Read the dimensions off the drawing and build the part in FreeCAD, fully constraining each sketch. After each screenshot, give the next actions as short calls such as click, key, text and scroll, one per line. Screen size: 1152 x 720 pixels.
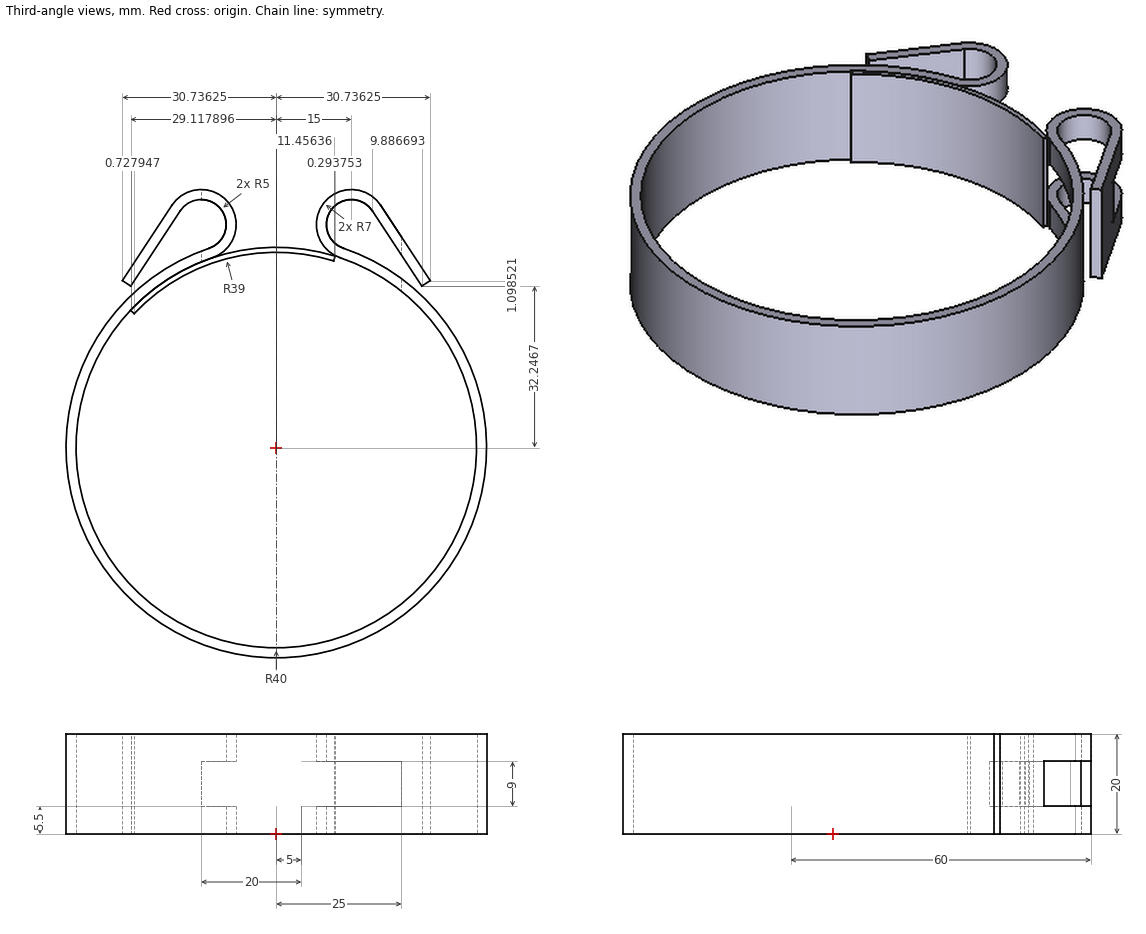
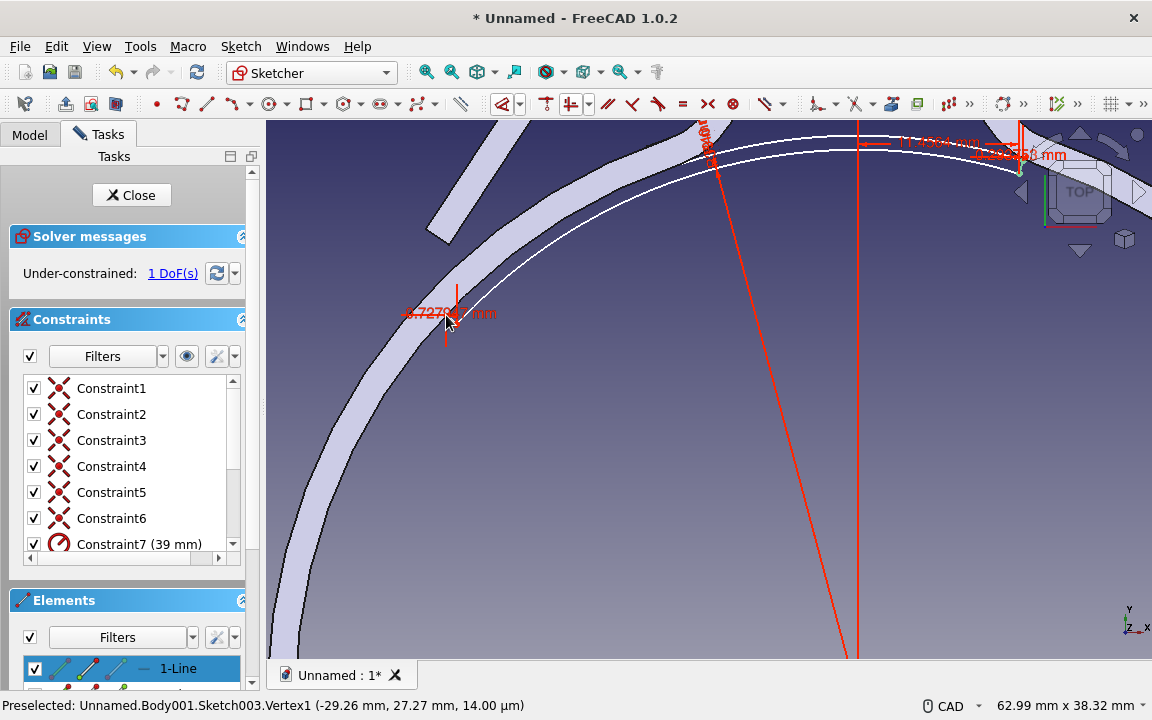
key(l)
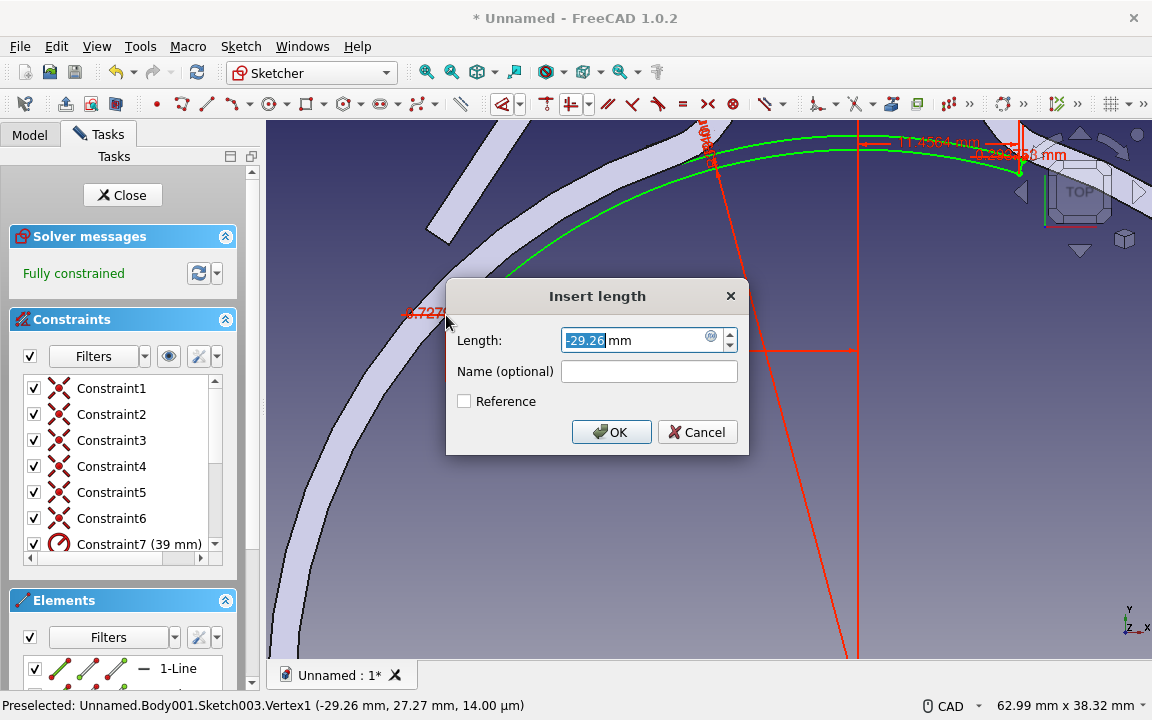
text(-29.117896)
key(Return)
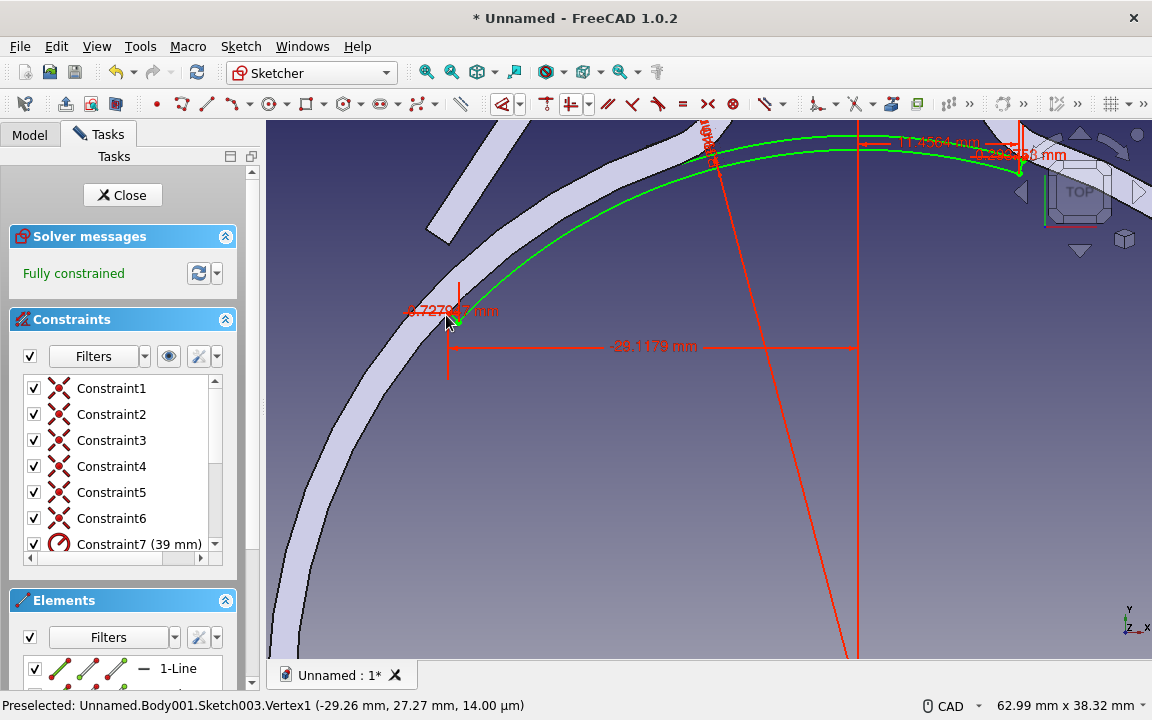
click(123, 195)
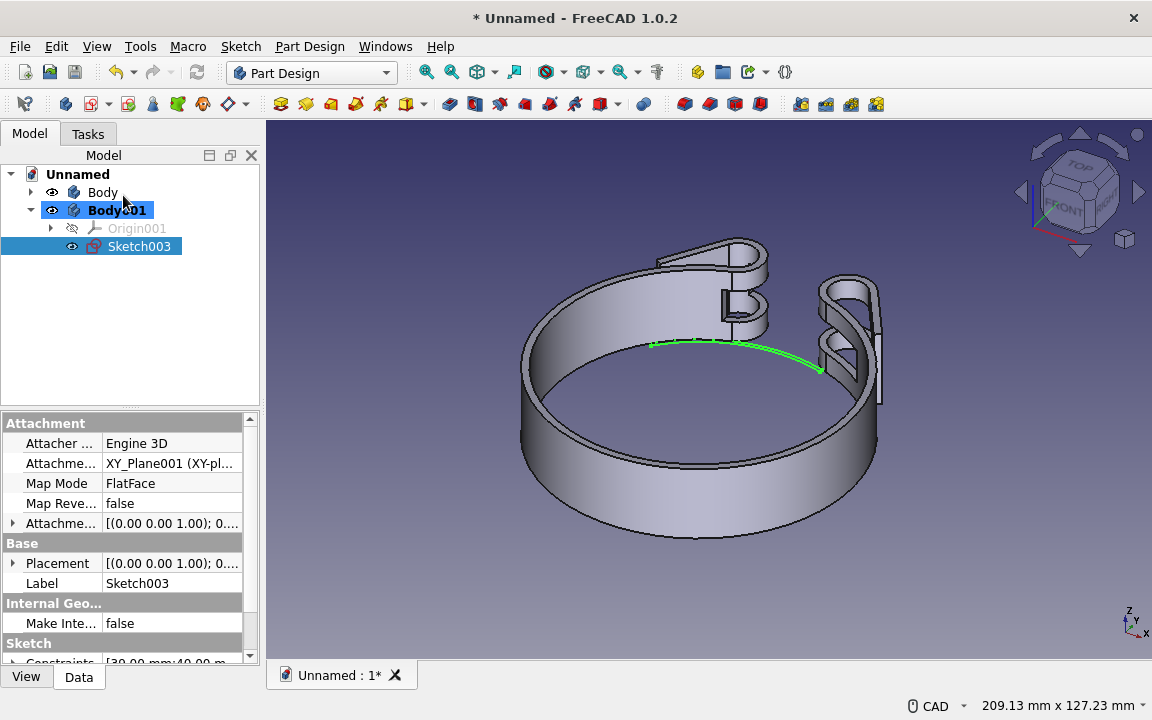
click(281, 104)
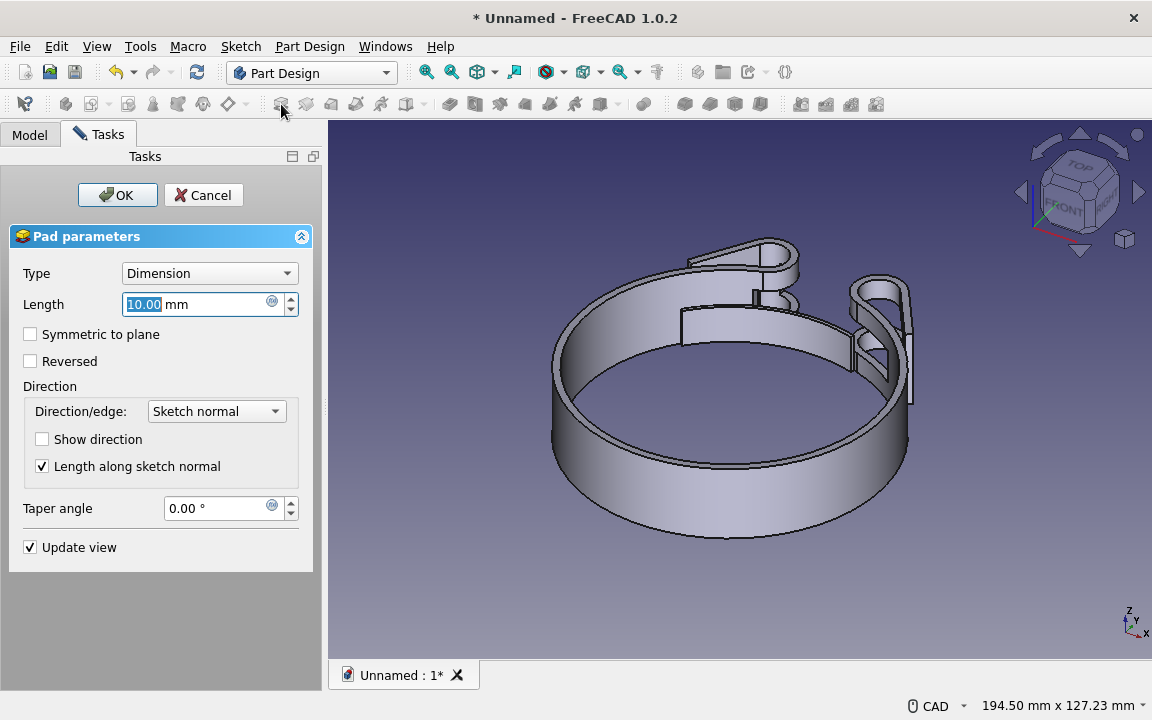
text(20)
key(Tab)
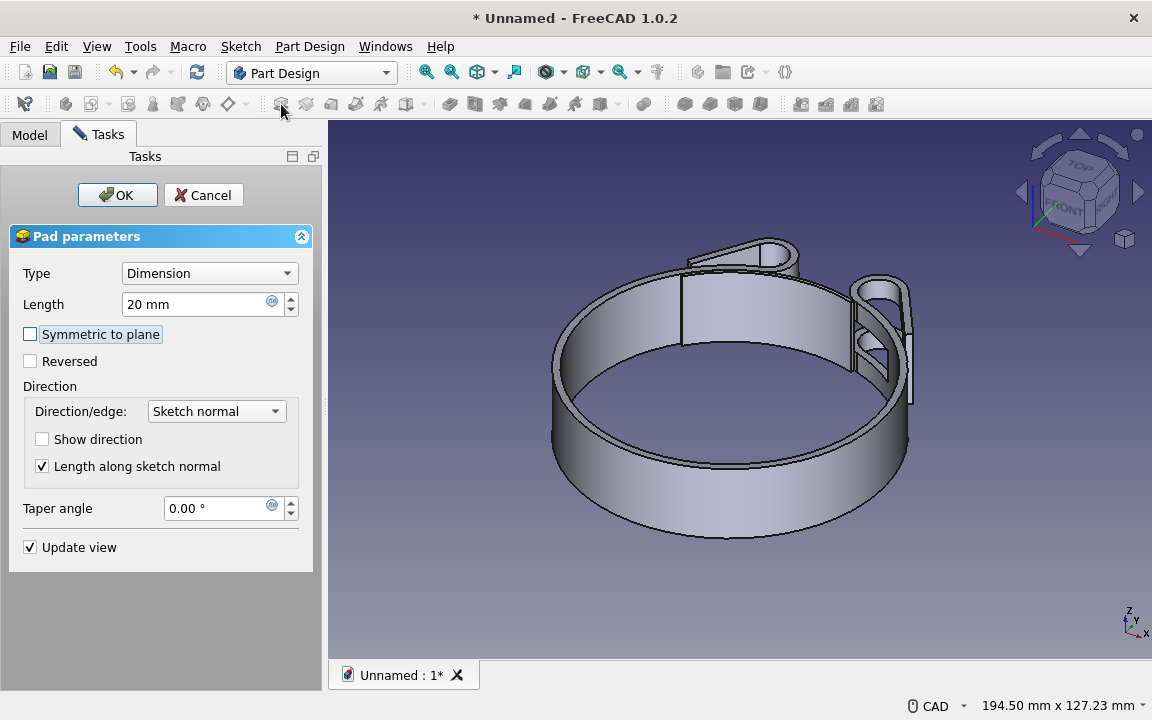
click(118, 195)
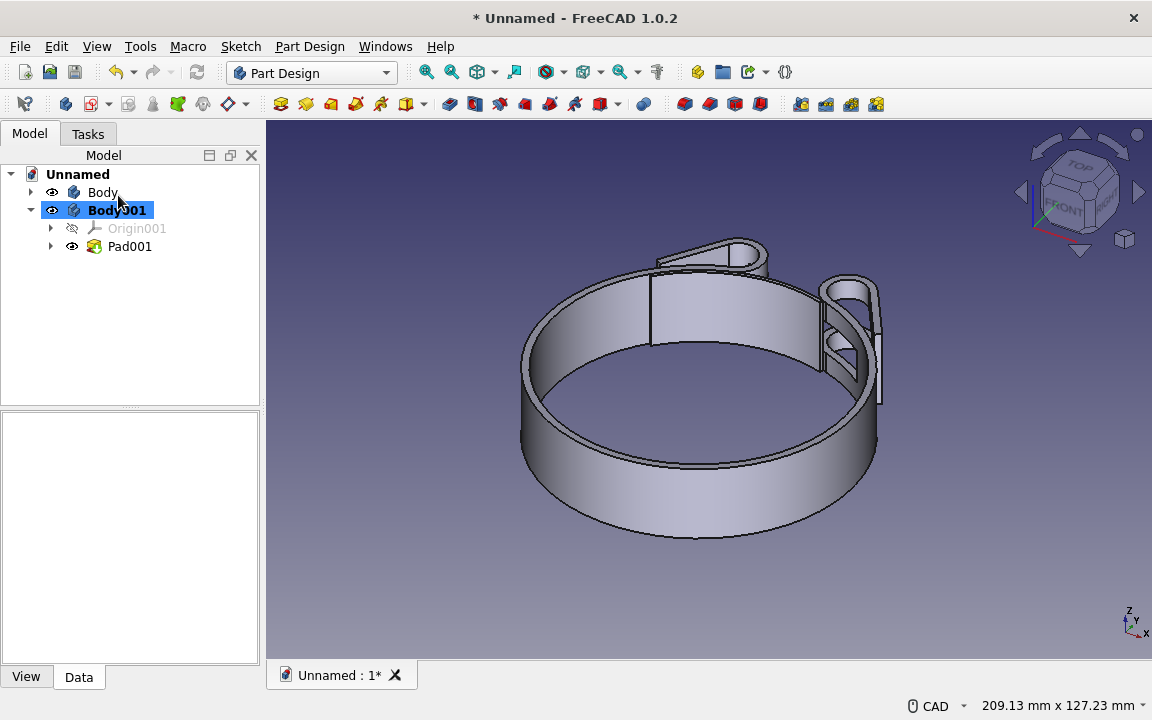
key(0)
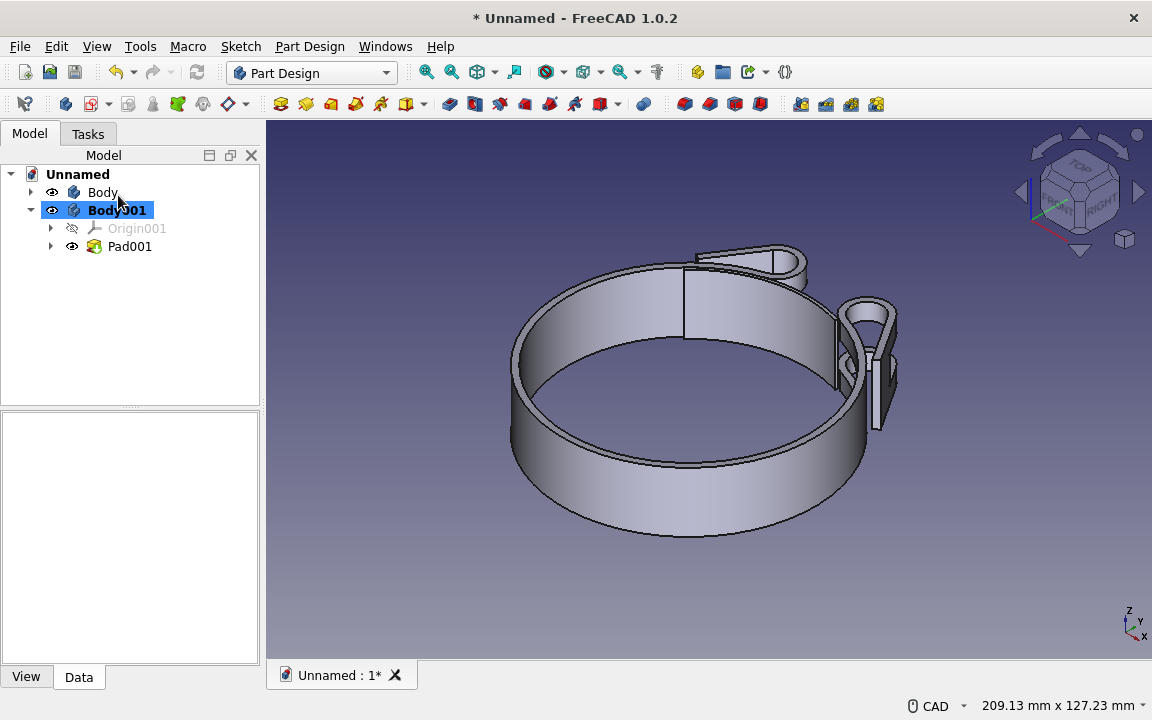
key(v)
key(f)